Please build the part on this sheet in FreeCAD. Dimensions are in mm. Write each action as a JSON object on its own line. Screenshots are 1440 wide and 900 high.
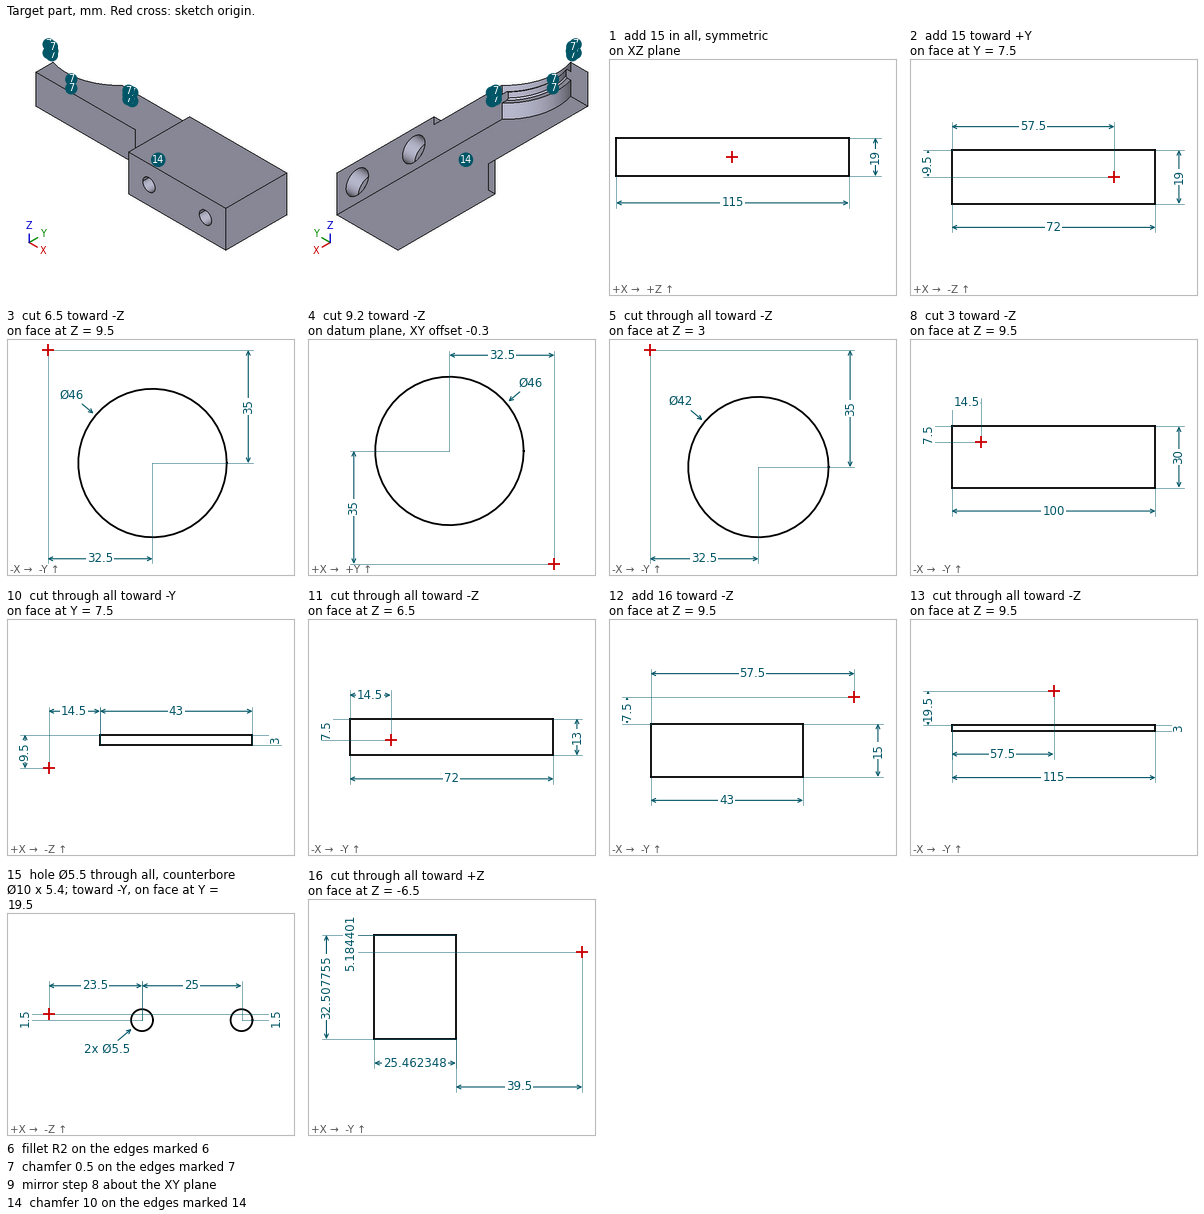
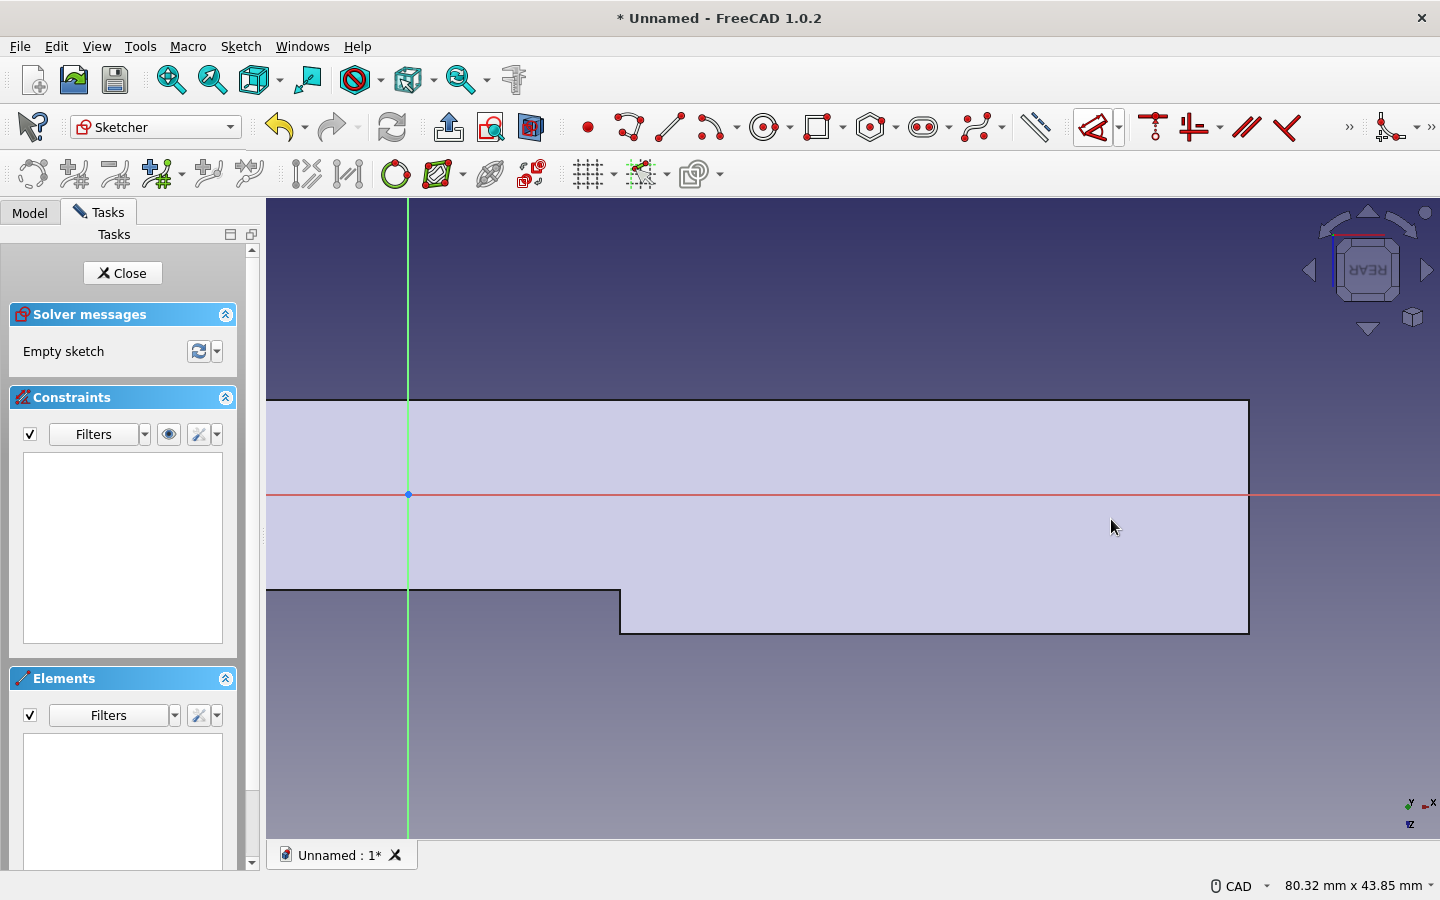
{"action": "left_click", "coordinate": [764, 128]}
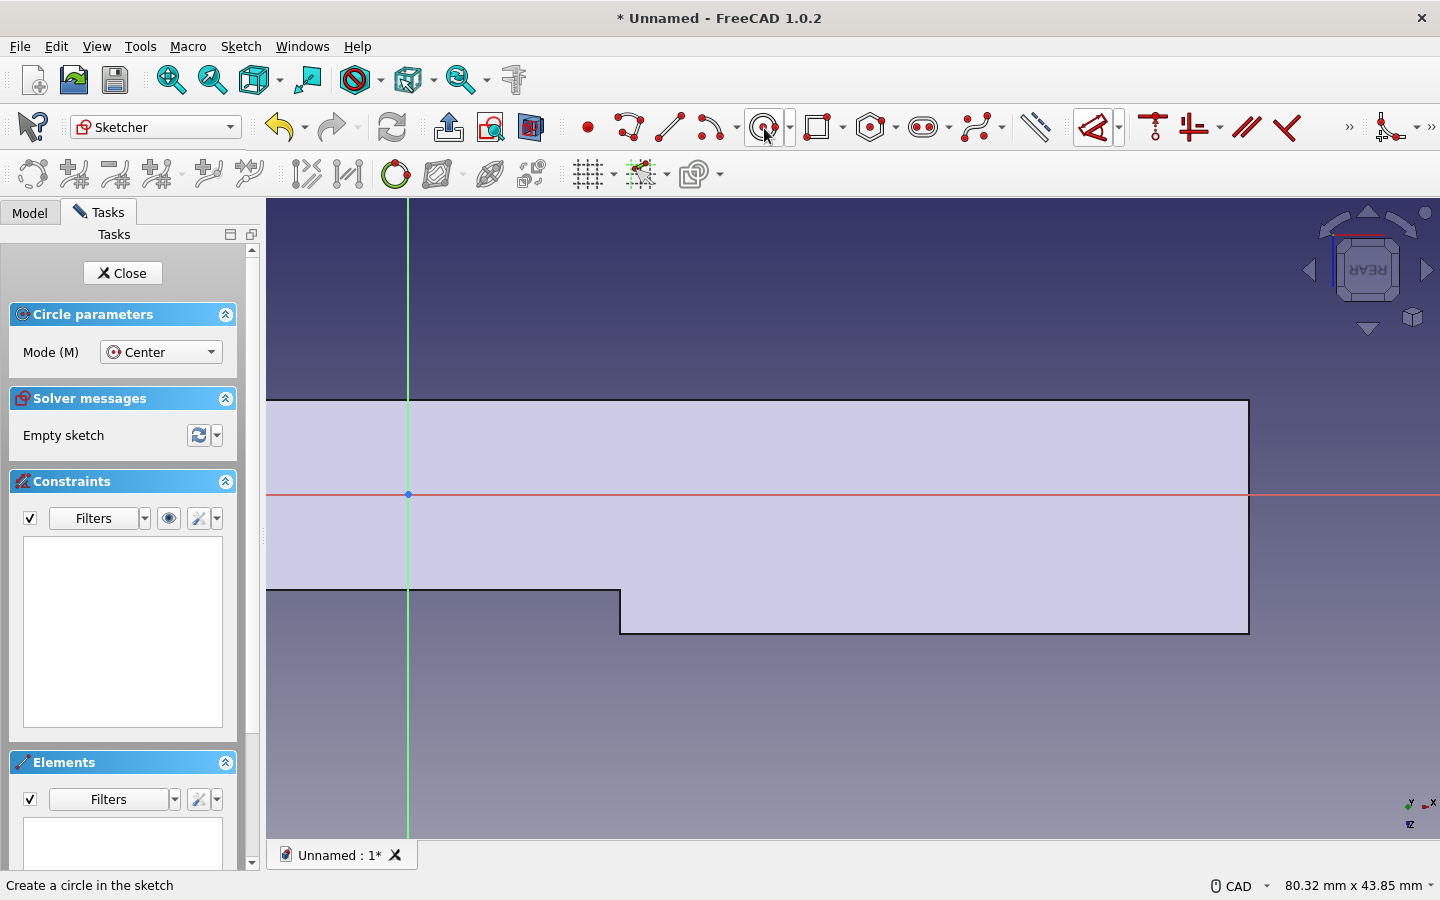
{"action": "left_click", "coordinate": [752, 517]}
{"action": "mouse_move", "coordinate": [780, 545]}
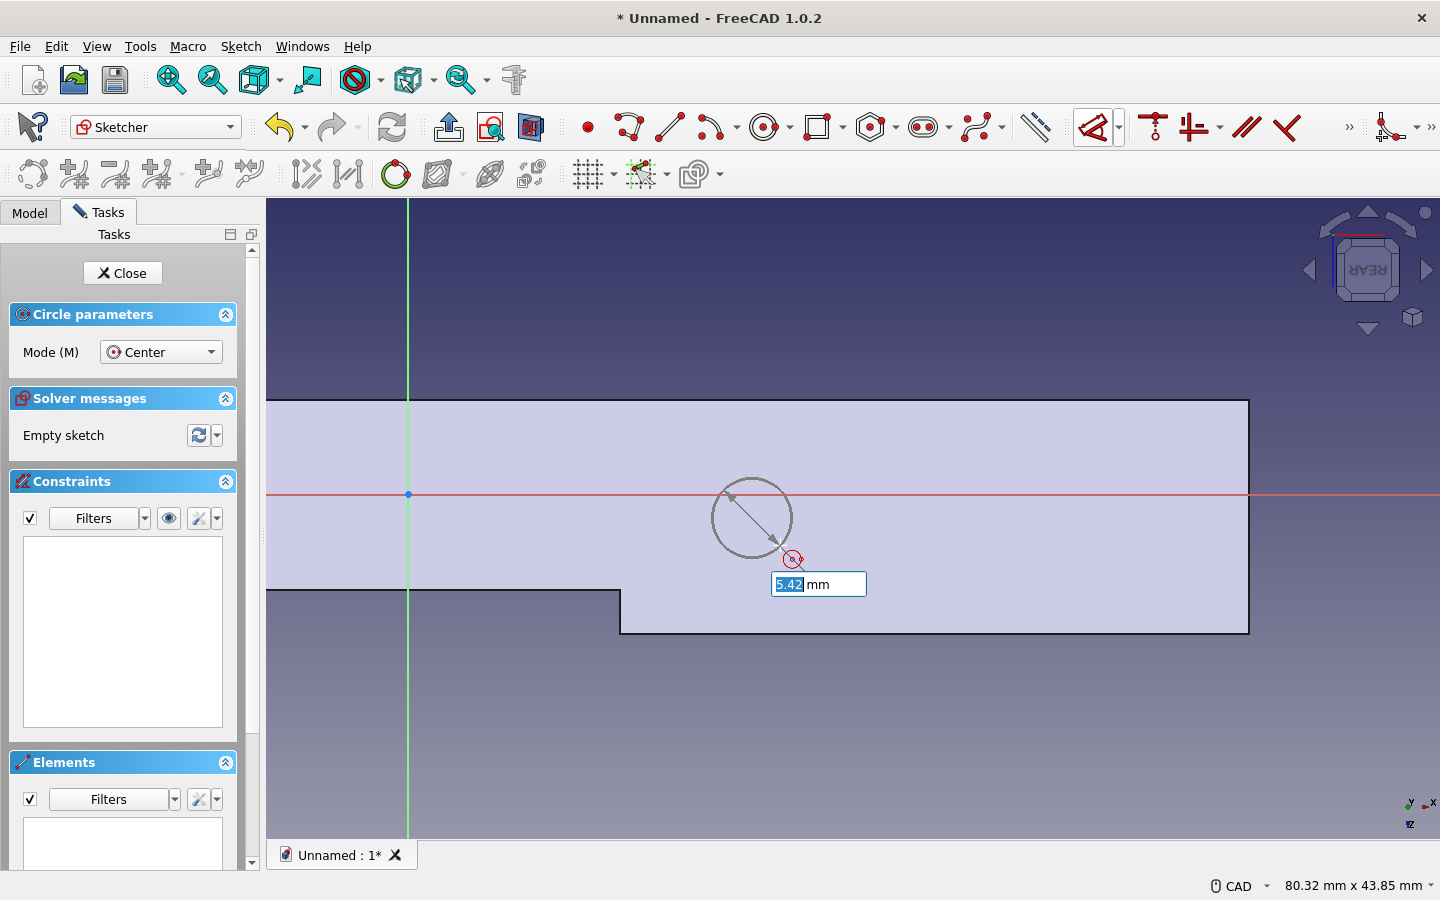
{"action": "type", "text": "5.5"}
{"action": "key", "text": "Return"}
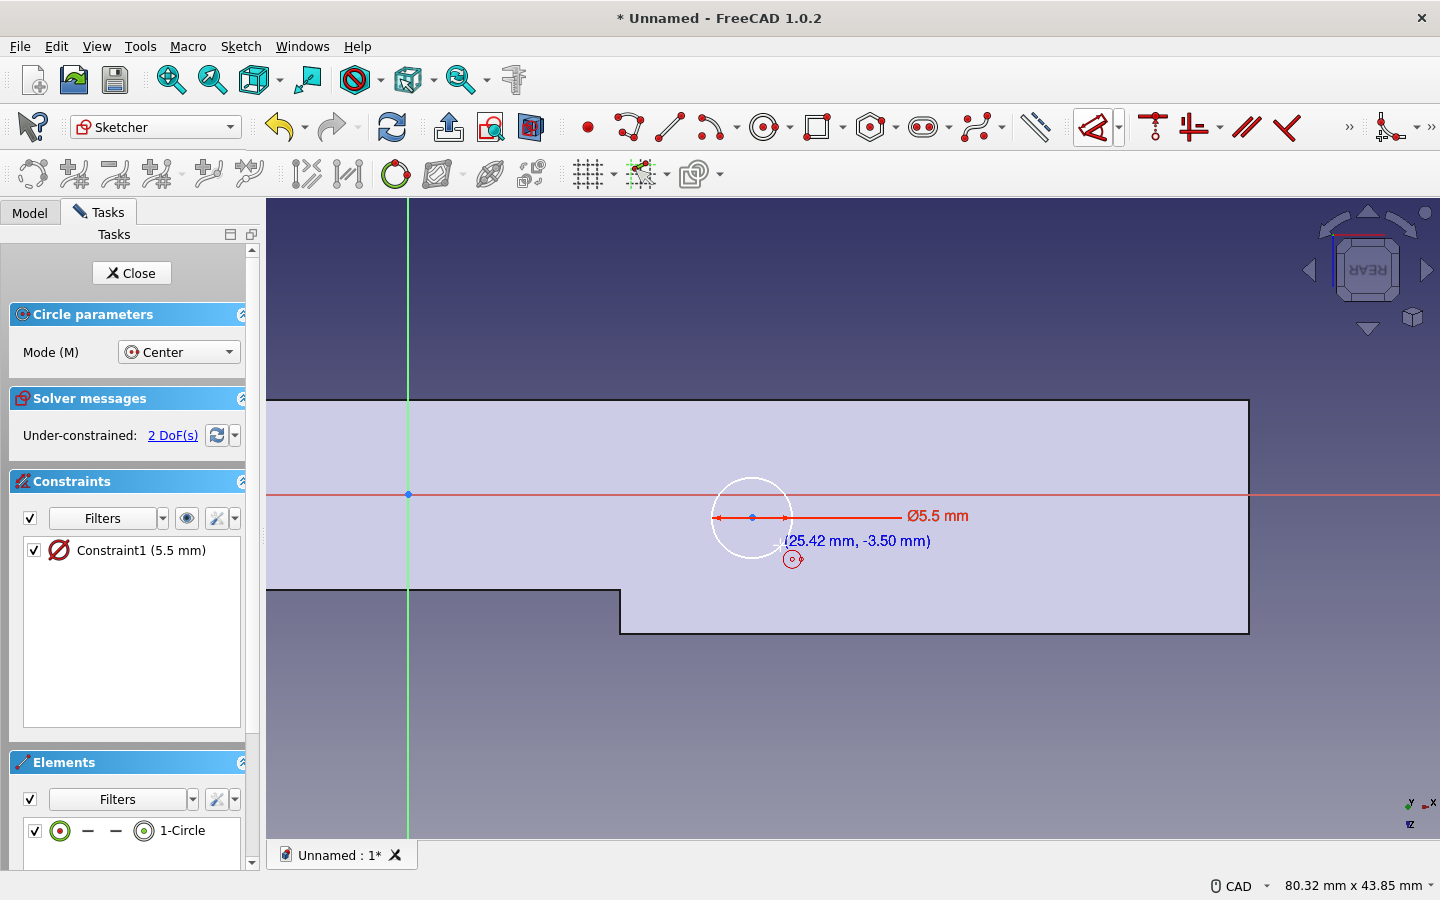
{"action": "left_click", "coordinate": [1117, 517]}
{"action": "mouse_move", "coordinate": [1146, 545]}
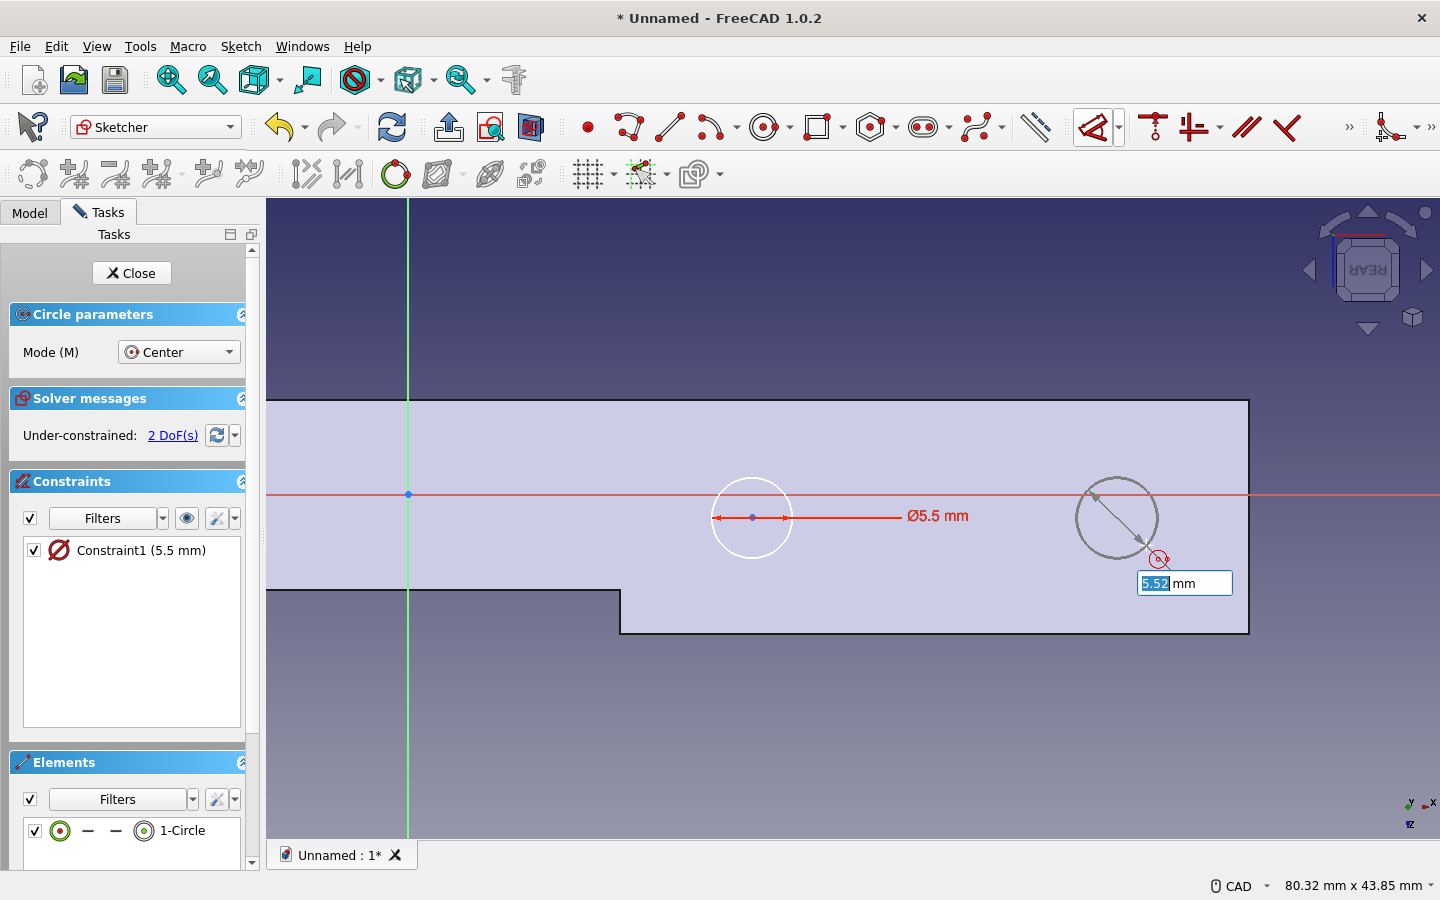
{"action": "type", "text": "5.5"}
{"action": "key", "text": "Return"}
{"action": "key", "text": "Escape"}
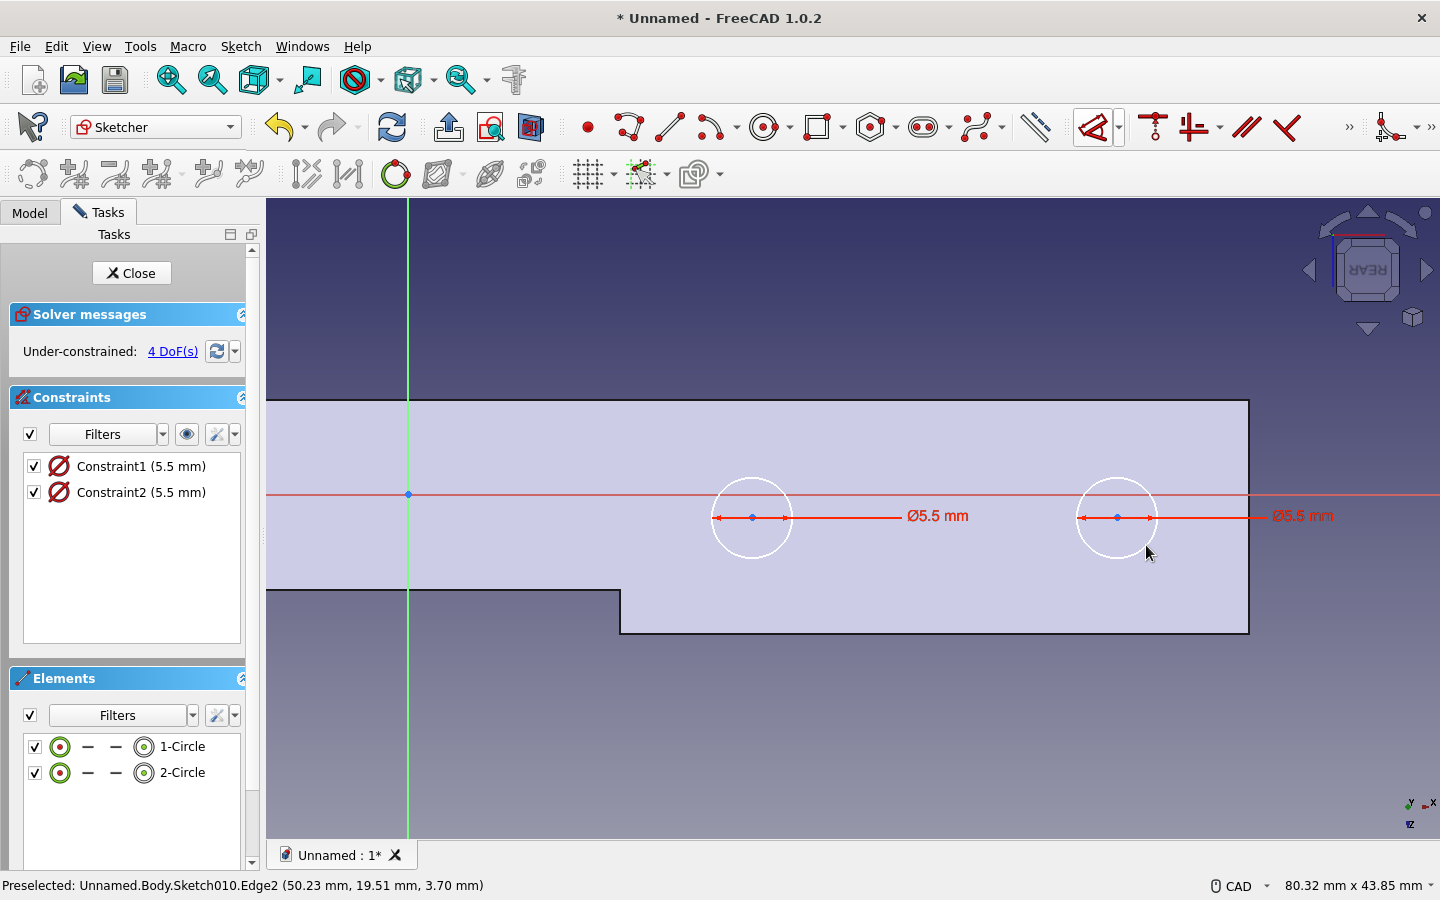
{"action": "scroll", "coordinate": [752, 518], "scroll_direction": "up", "scroll_amount": 3}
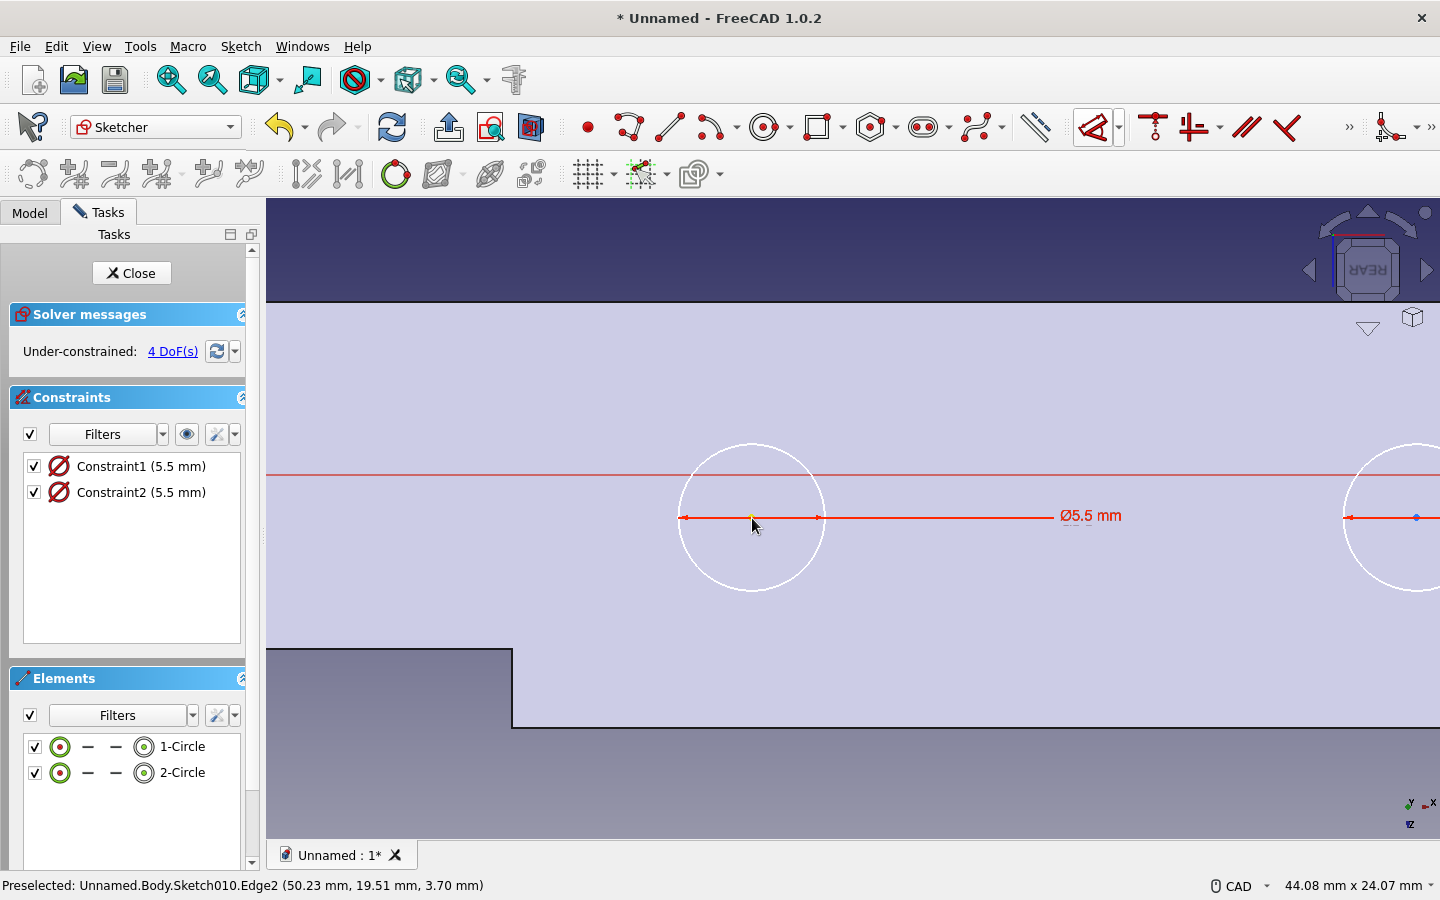
{"action": "left_click", "coordinate": [752, 518]}